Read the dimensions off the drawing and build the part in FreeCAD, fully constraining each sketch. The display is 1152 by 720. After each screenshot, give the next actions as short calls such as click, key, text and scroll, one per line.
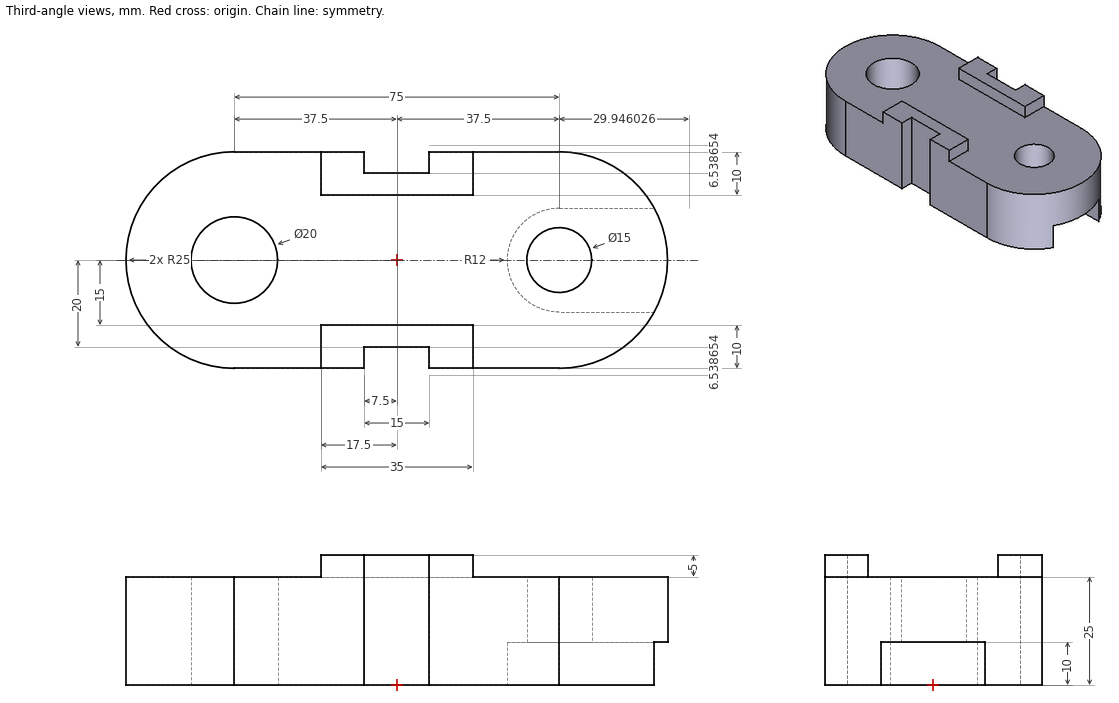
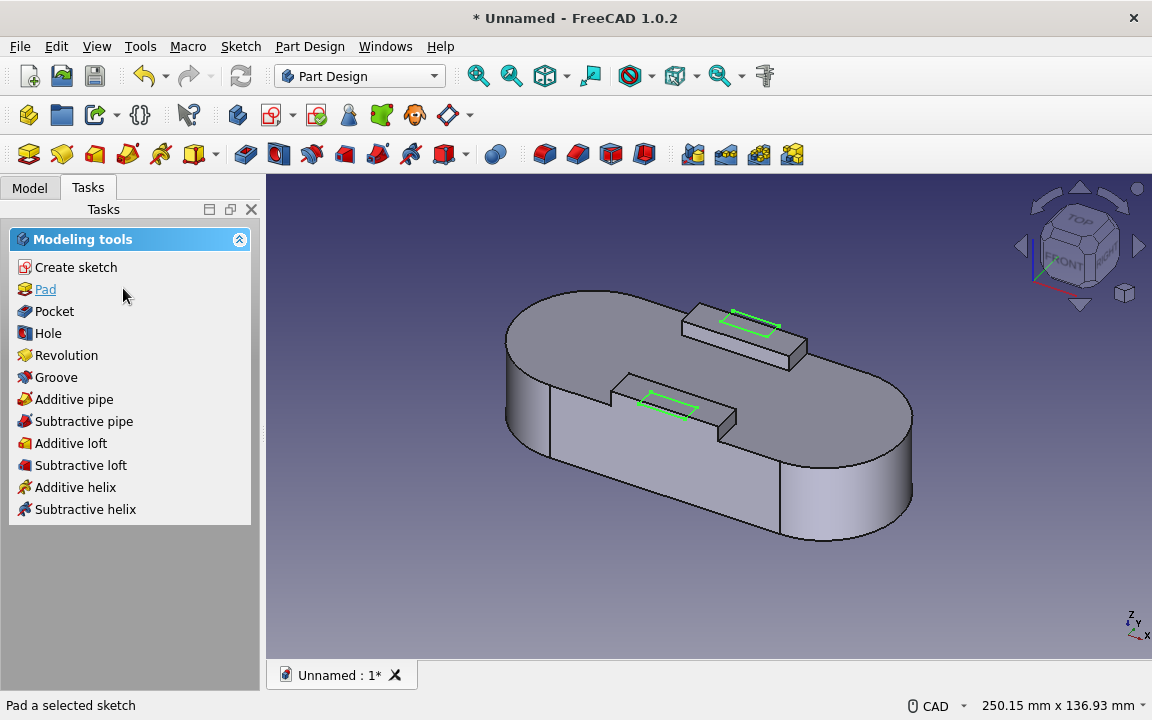
click(246, 154)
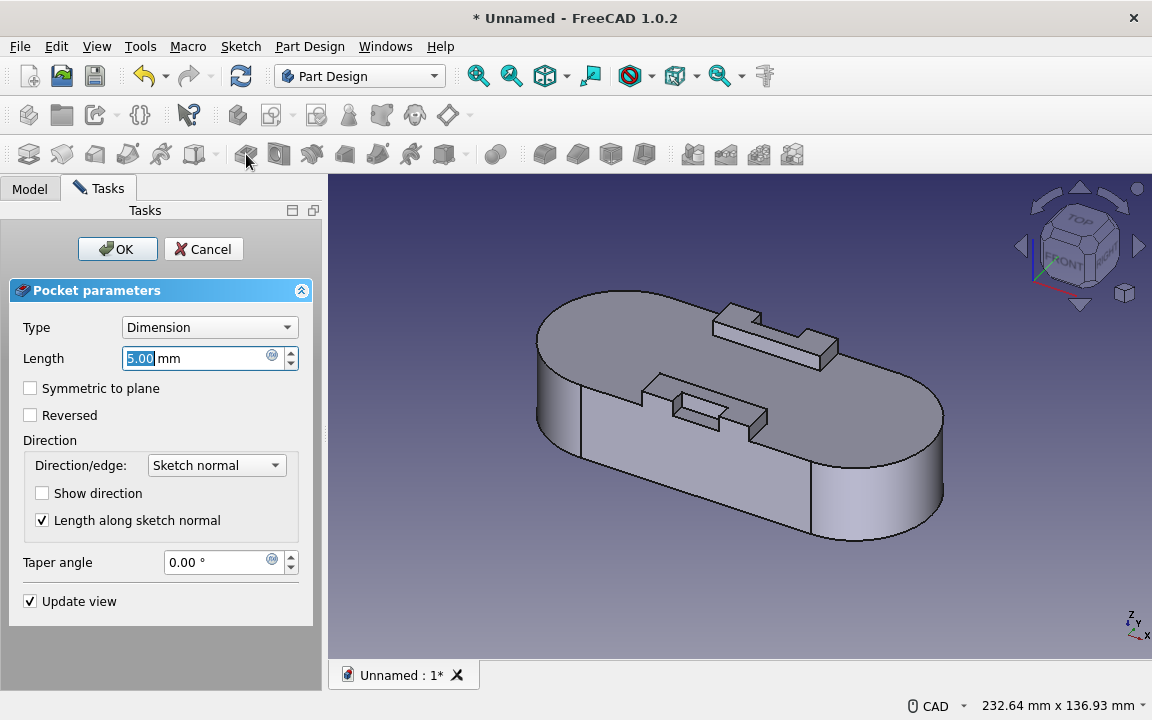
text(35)
key(Tab)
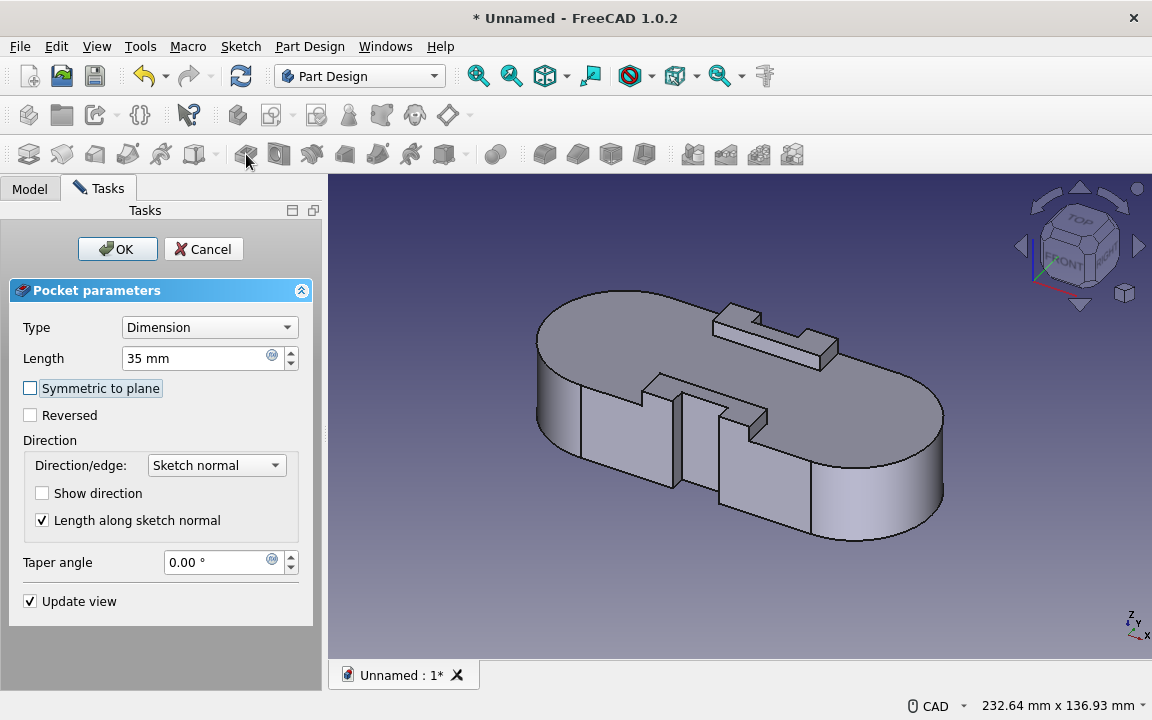
click(118, 249)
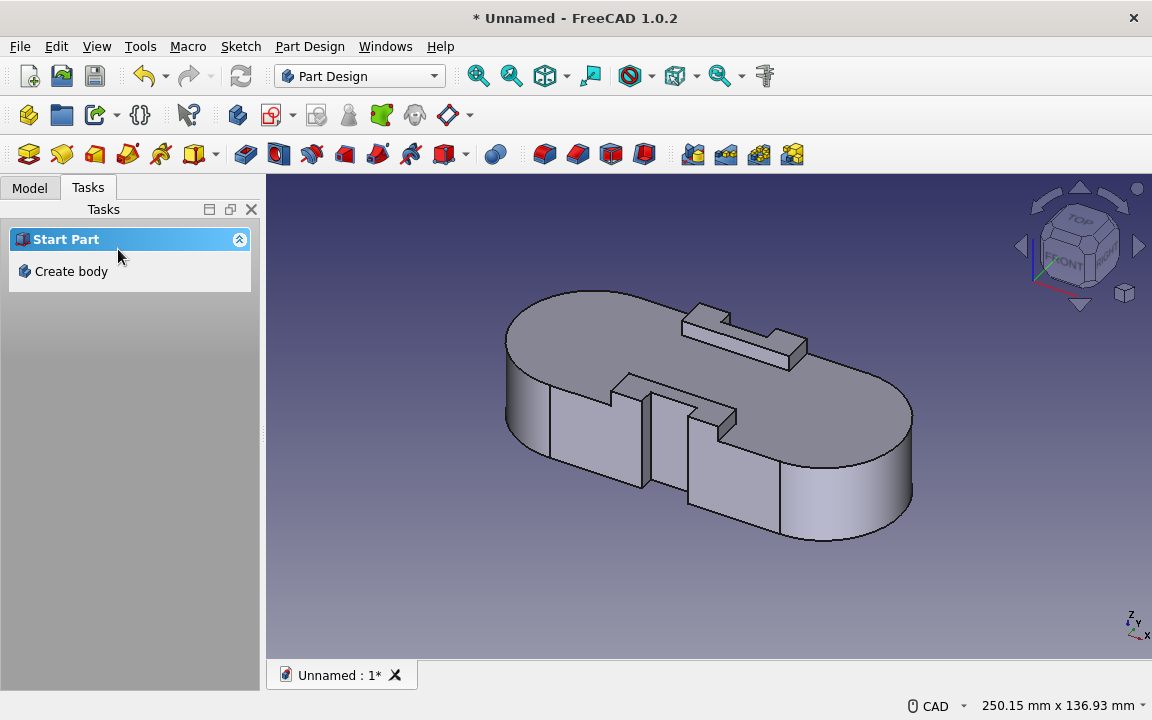
key(5)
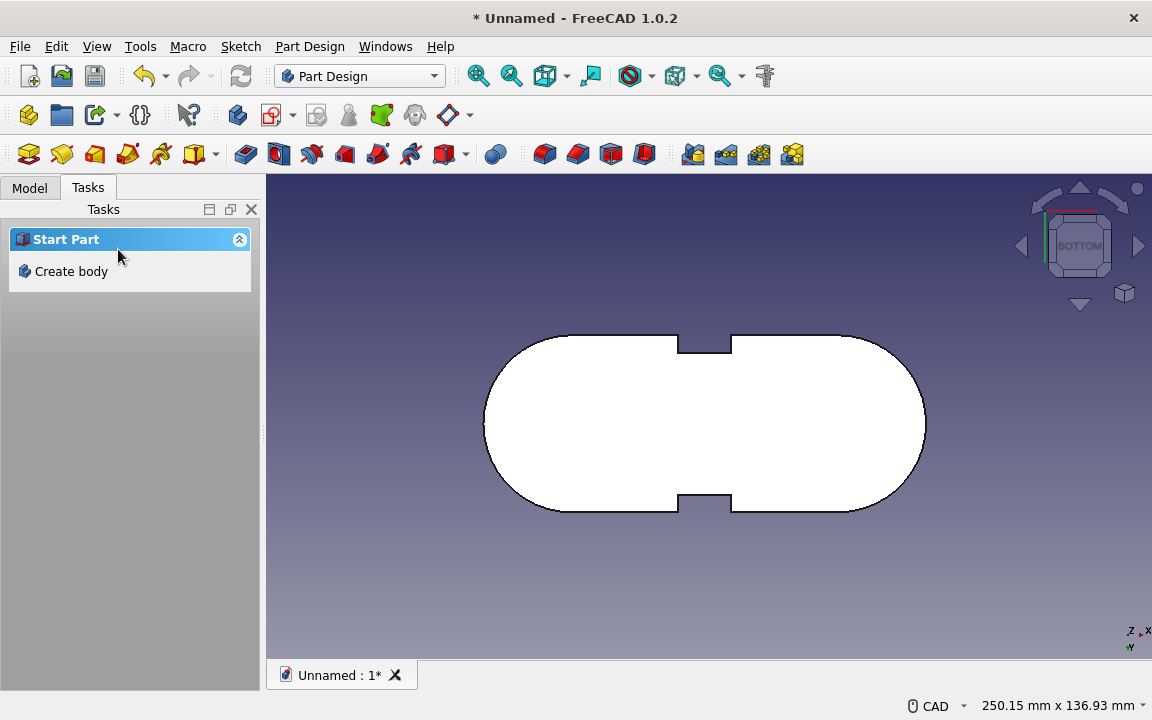
click(831, 423)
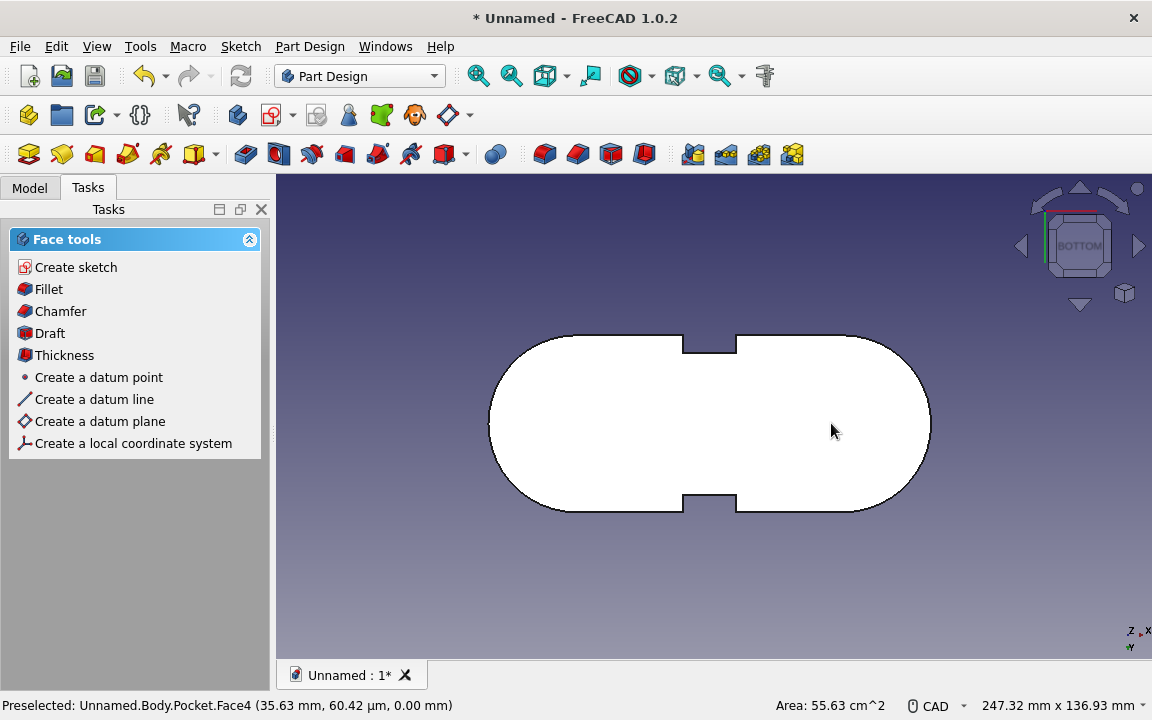
click(270, 116)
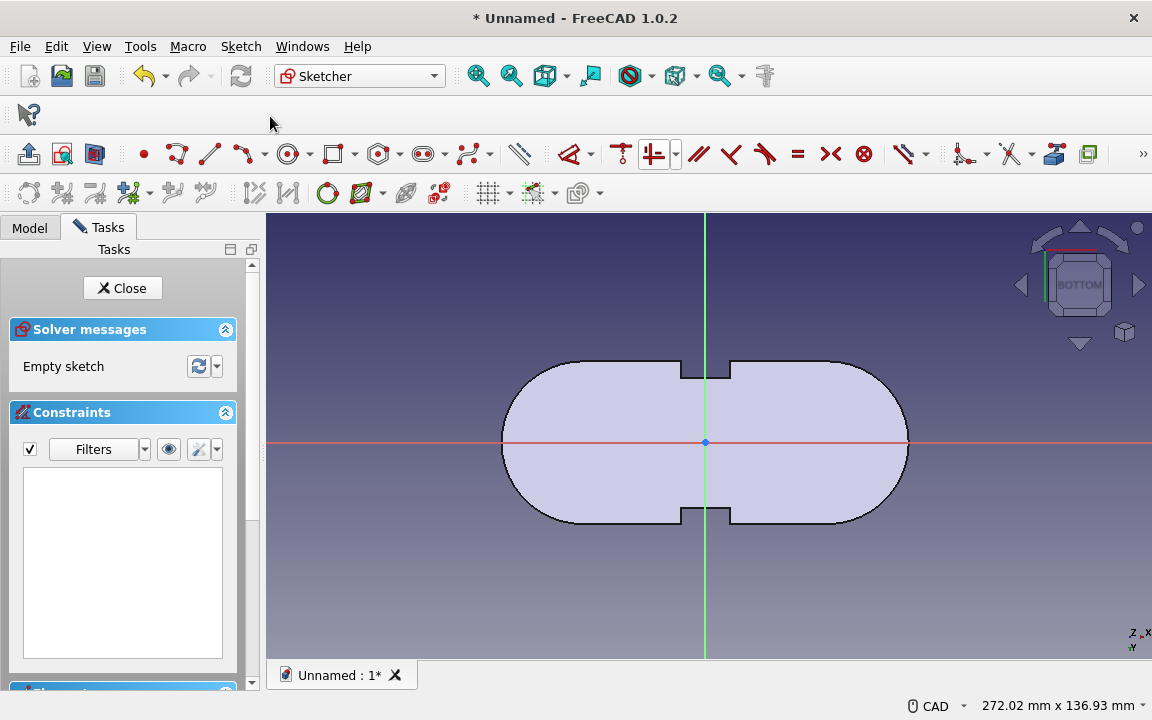
scroll(957, 448, up, 4)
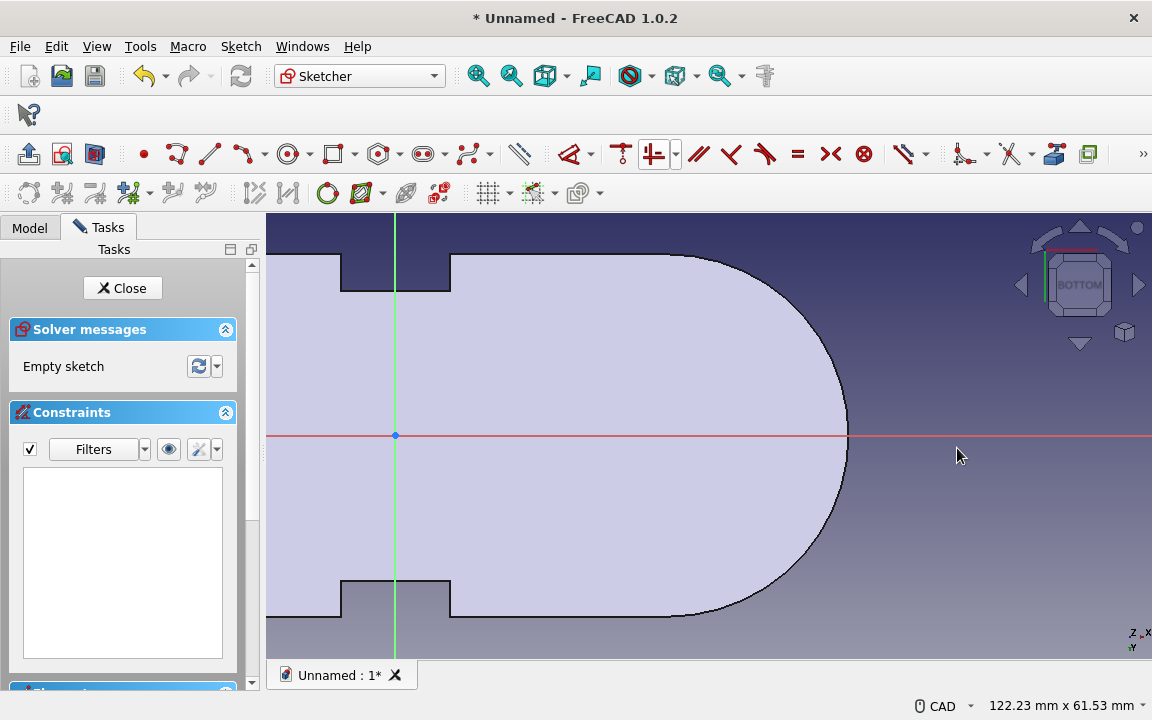
click(177, 154)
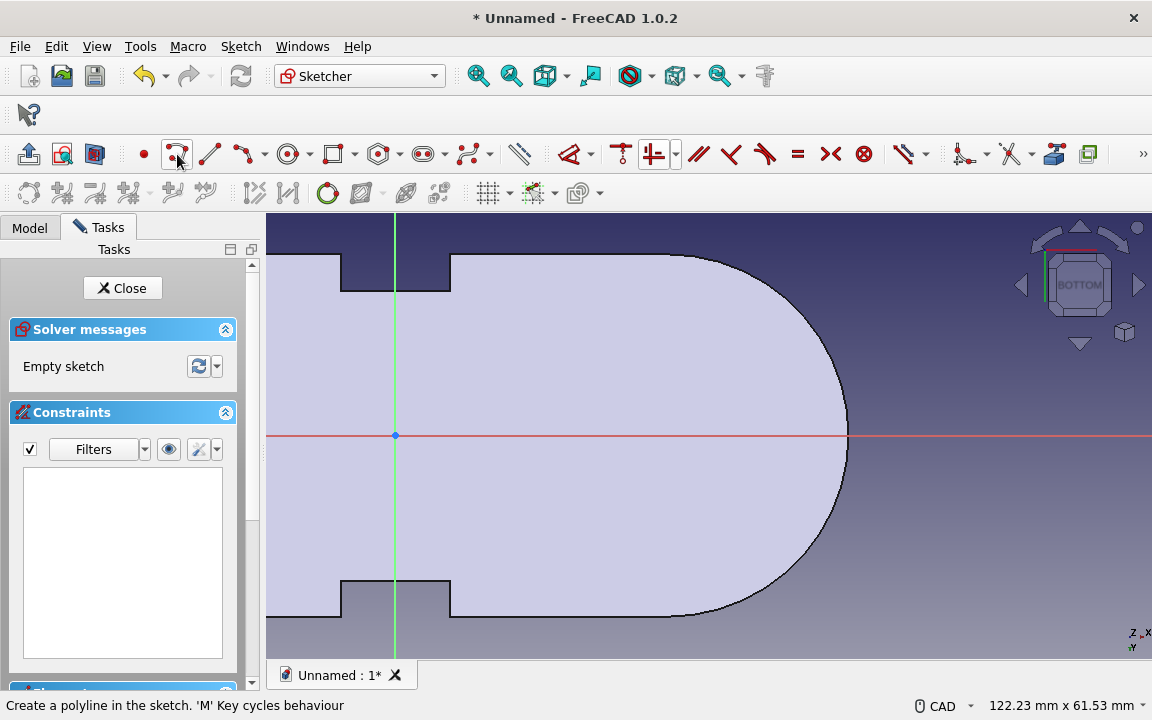
click(667, 523)
click(884, 523)
click(884, 349)
click(667, 349)
right_click(667, 349)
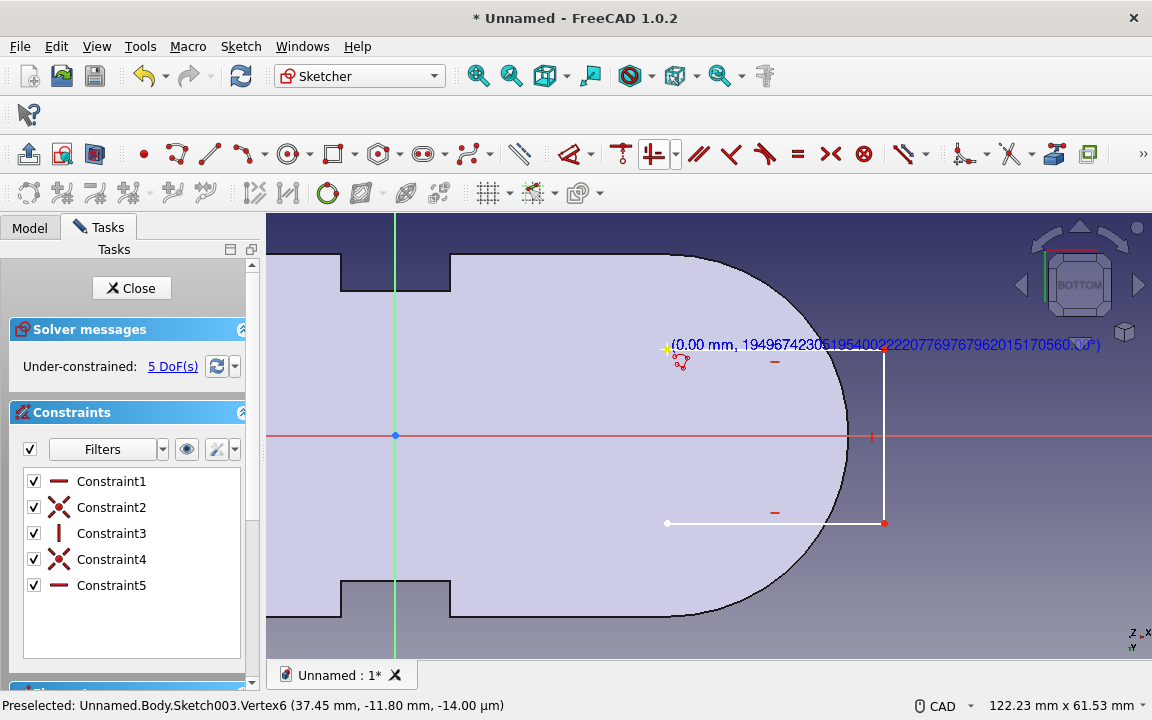
click(242, 154)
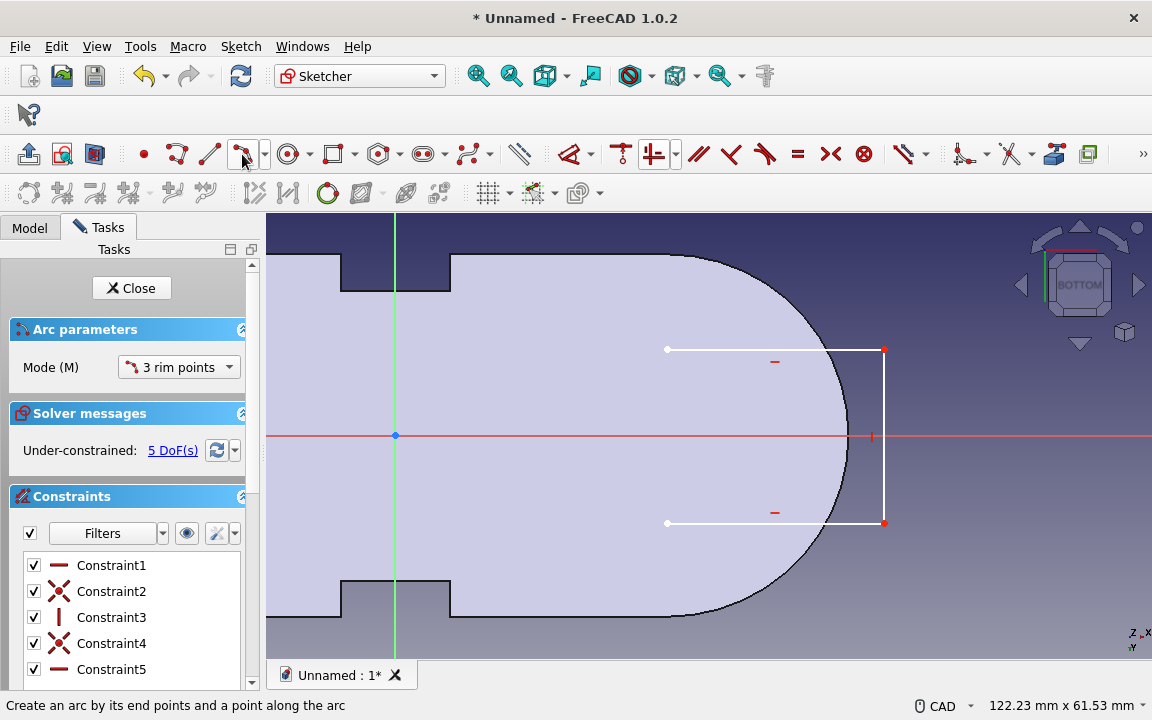
click(667, 350)
click(667, 524)
click(585, 409)
key(Escape)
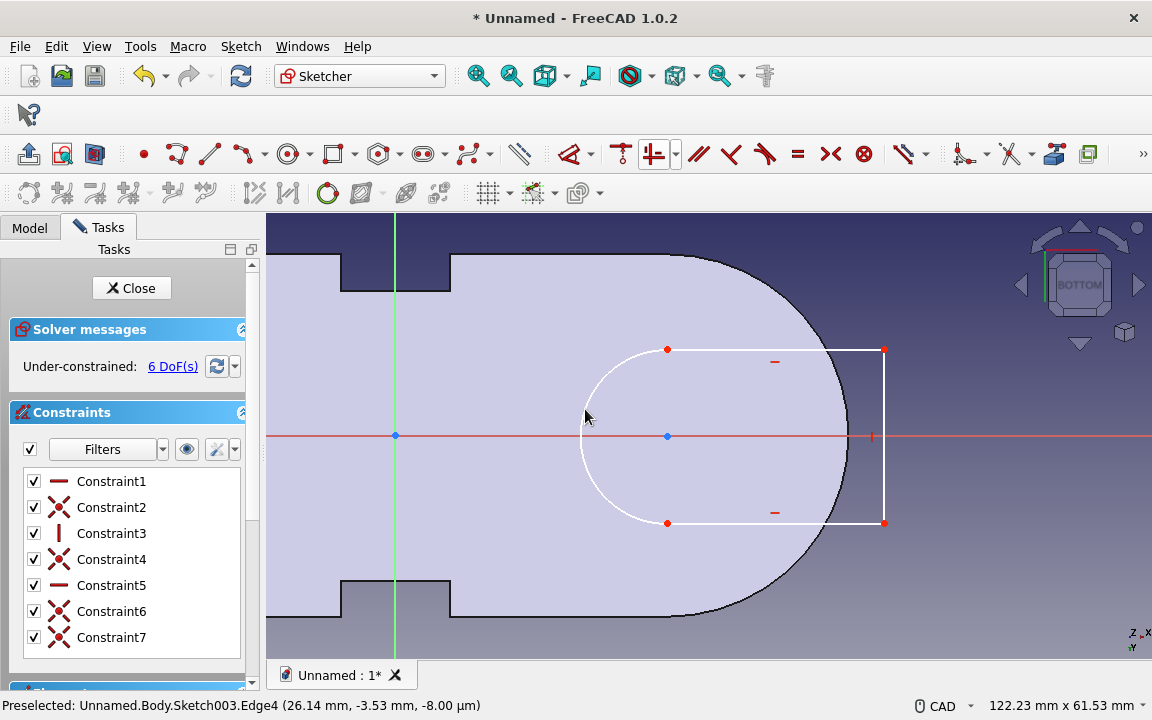
click(732, 524)